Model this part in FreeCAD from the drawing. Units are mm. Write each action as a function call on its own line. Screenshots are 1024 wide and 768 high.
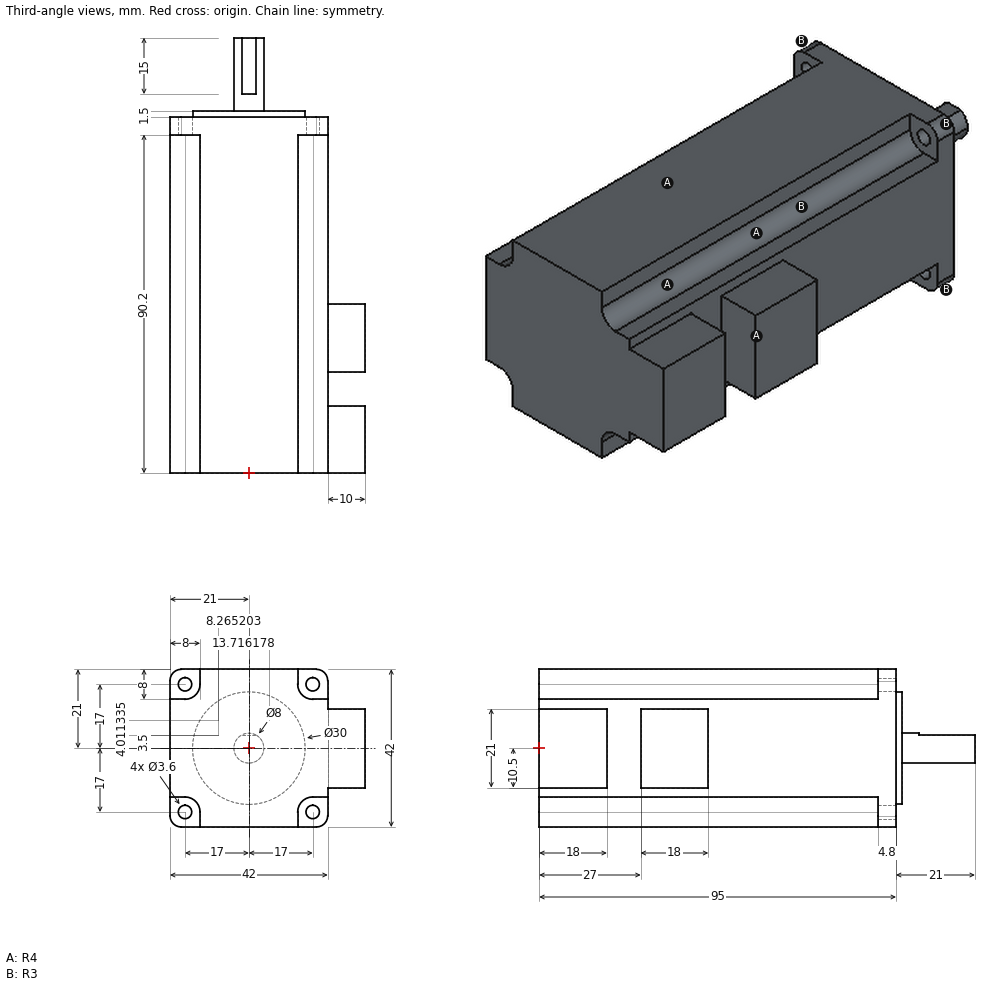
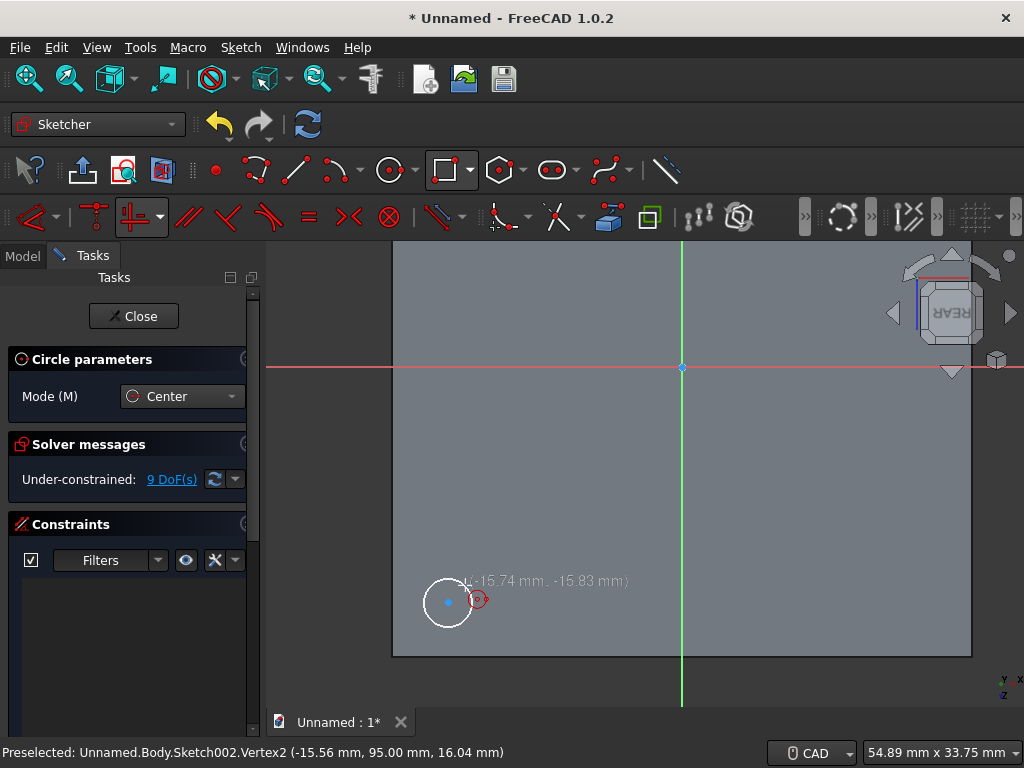
scroll(448, 604, down, 3)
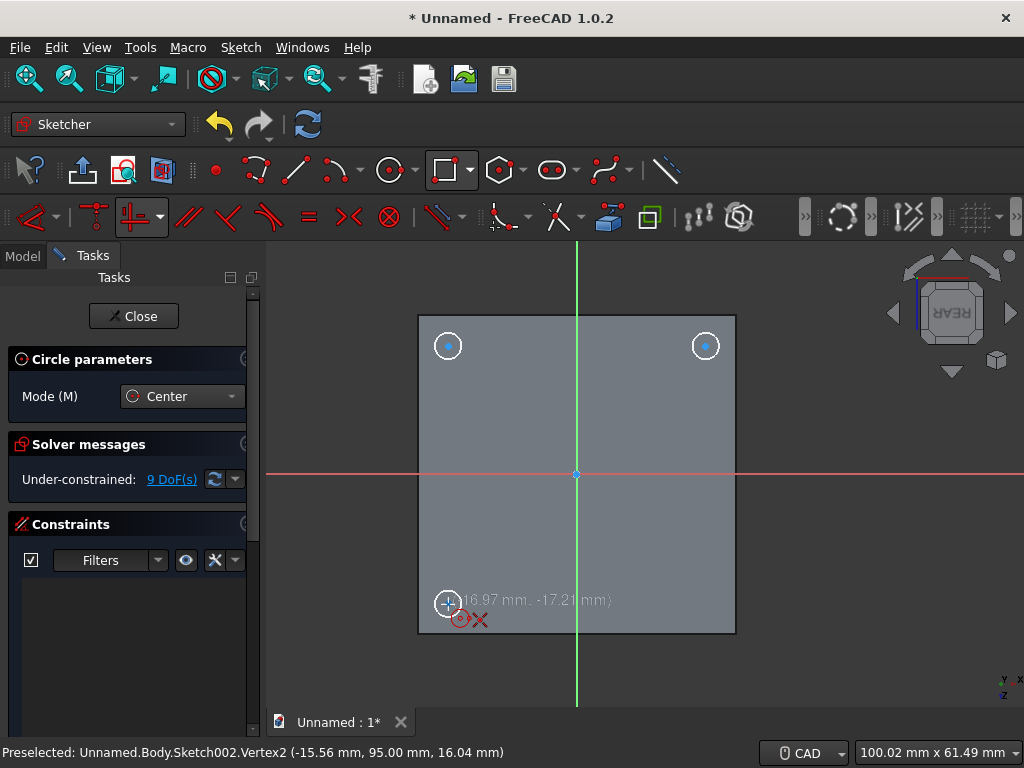
scroll(706, 603, up, 3)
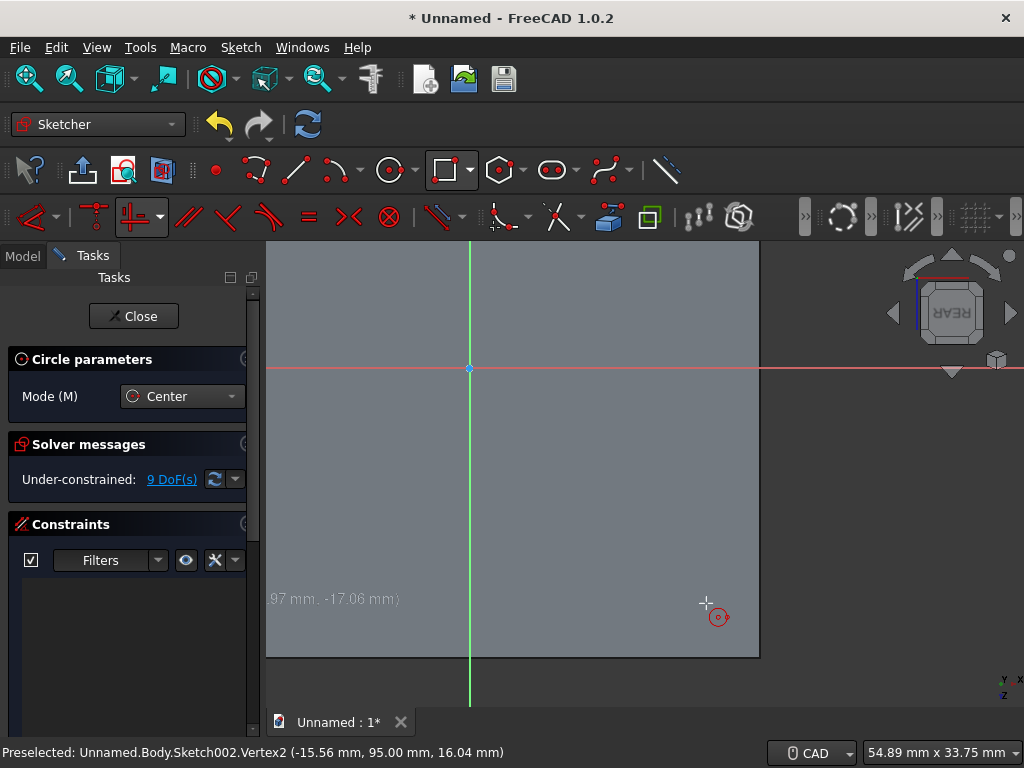
click(705, 603)
click(722, 585)
key(Escape)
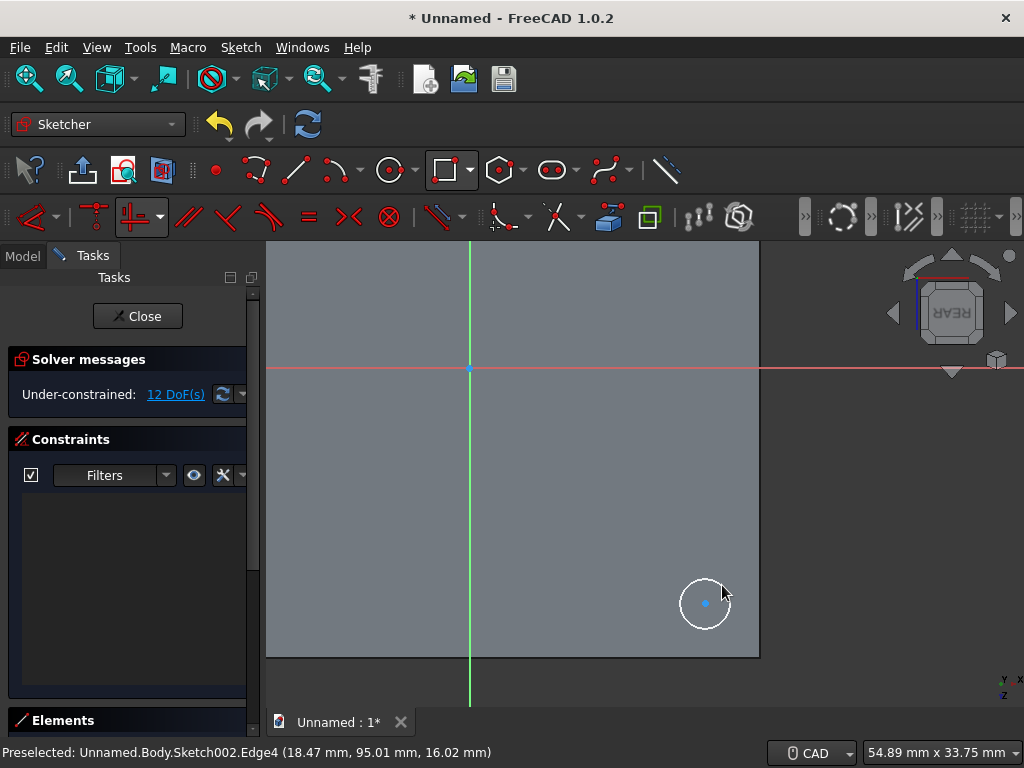
scroll(706, 603, down, 3)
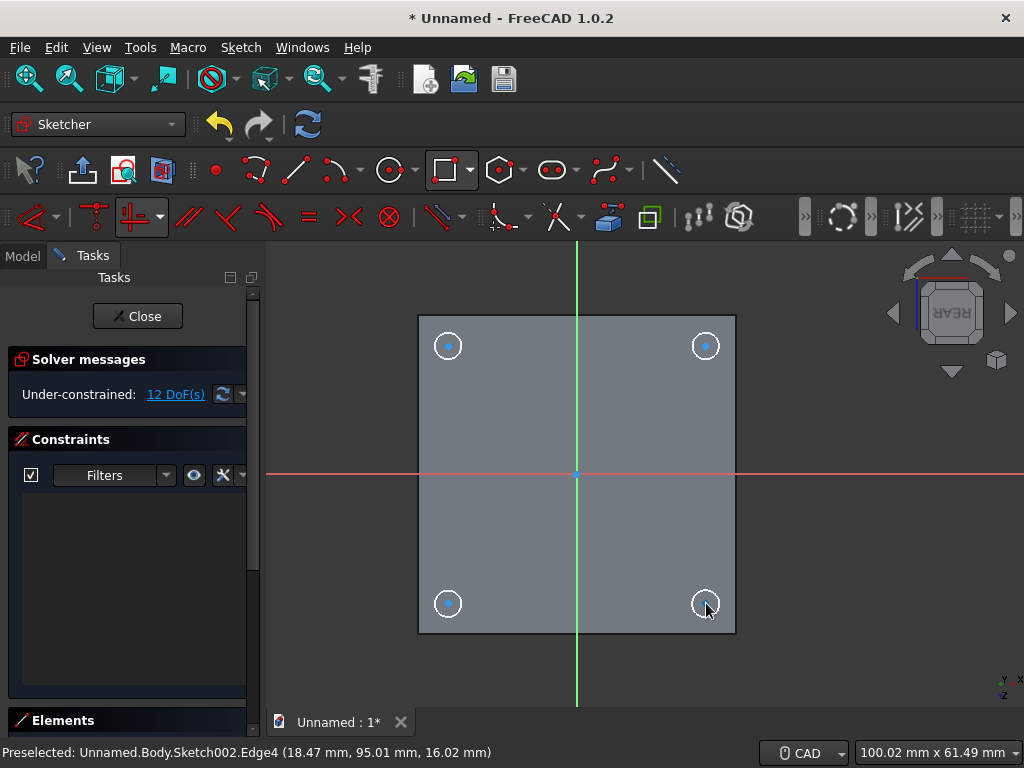
click(457, 337)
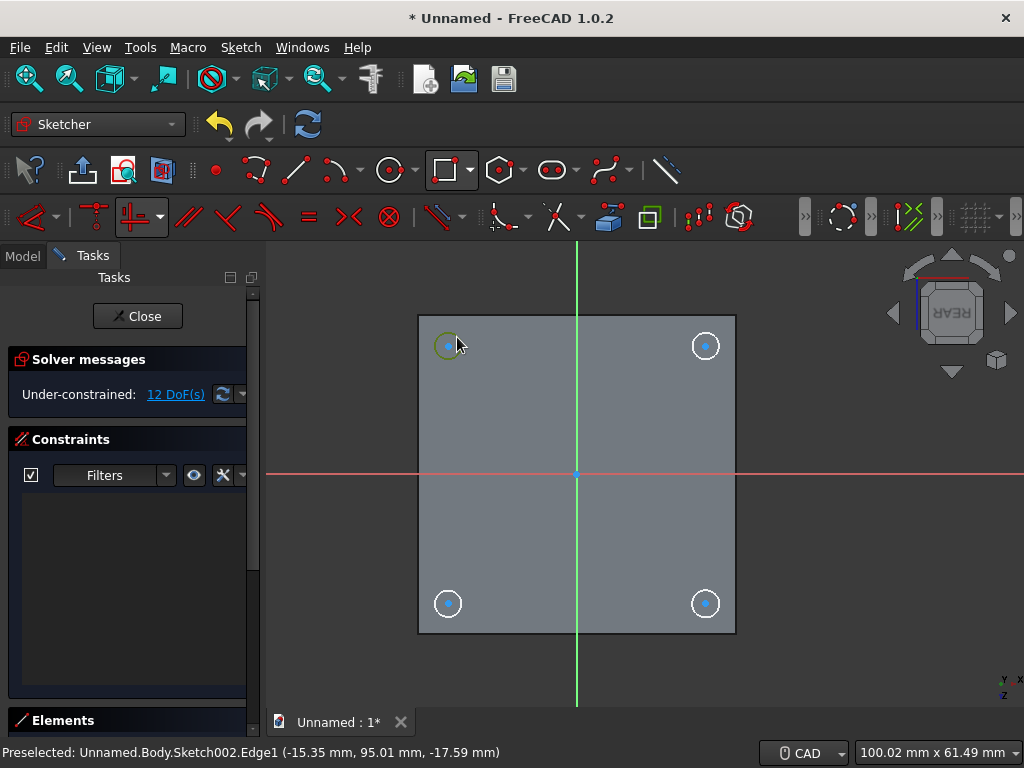
click(715, 337)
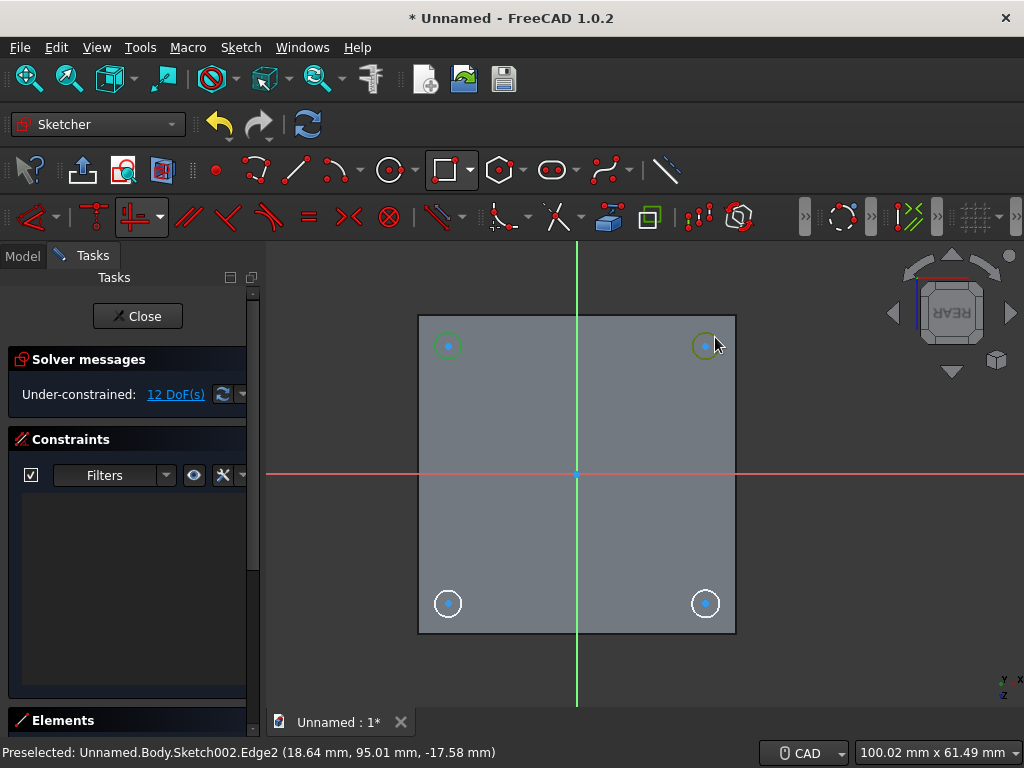
click(457, 594)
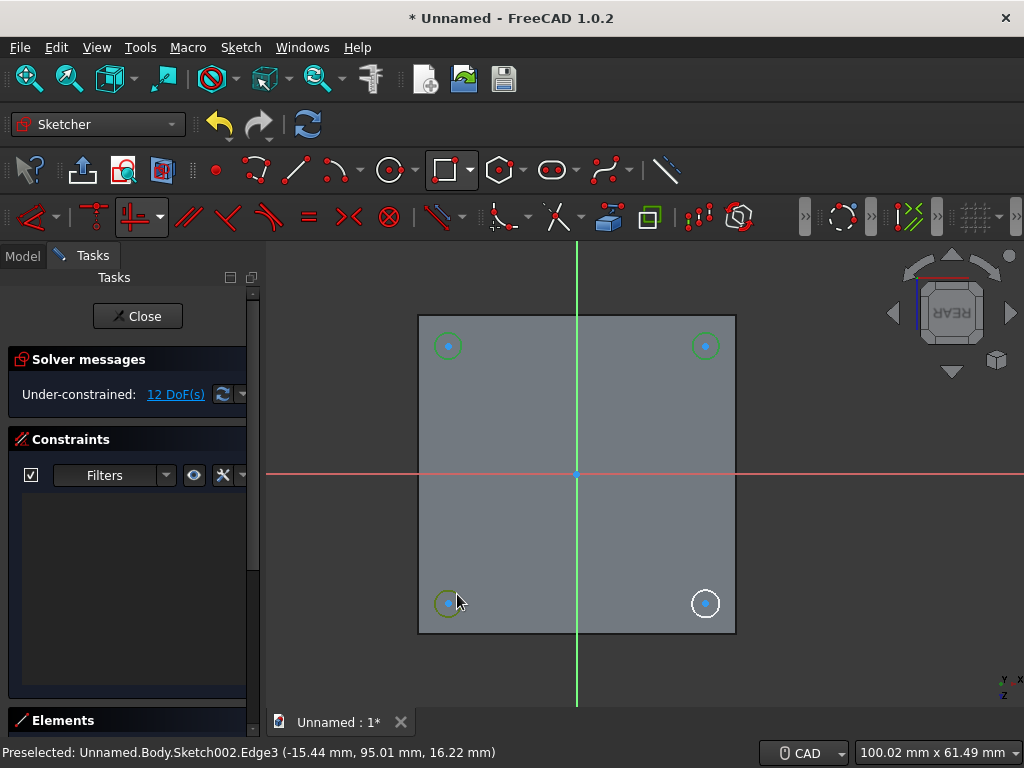
click(715, 594)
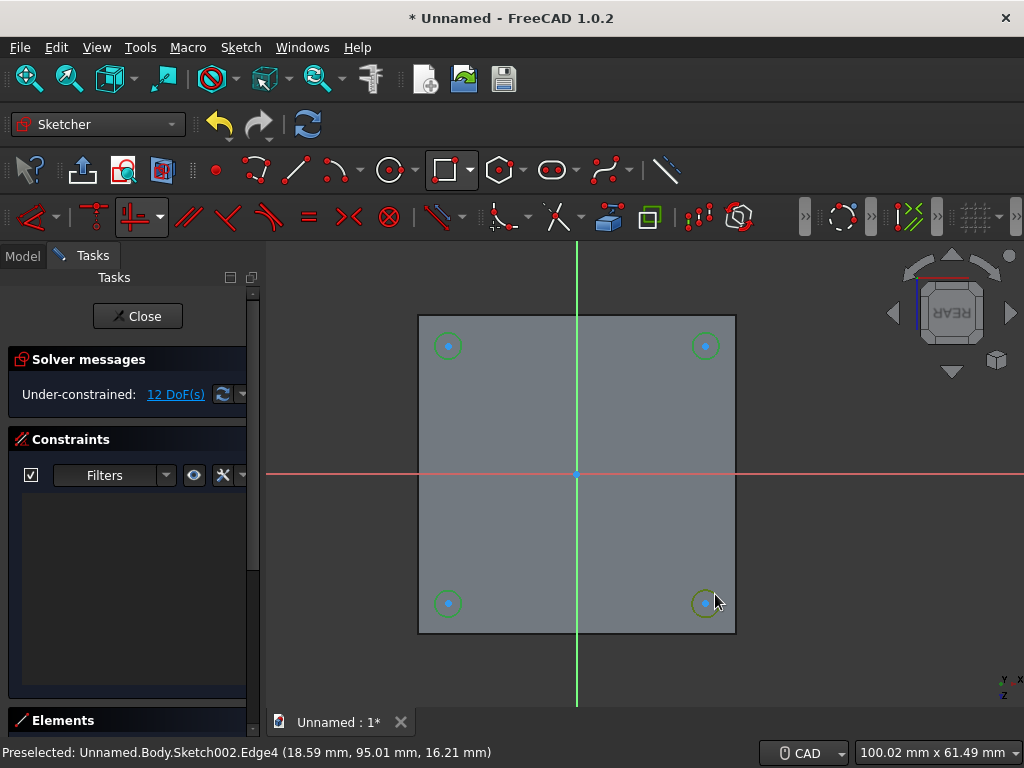
click(310, 218)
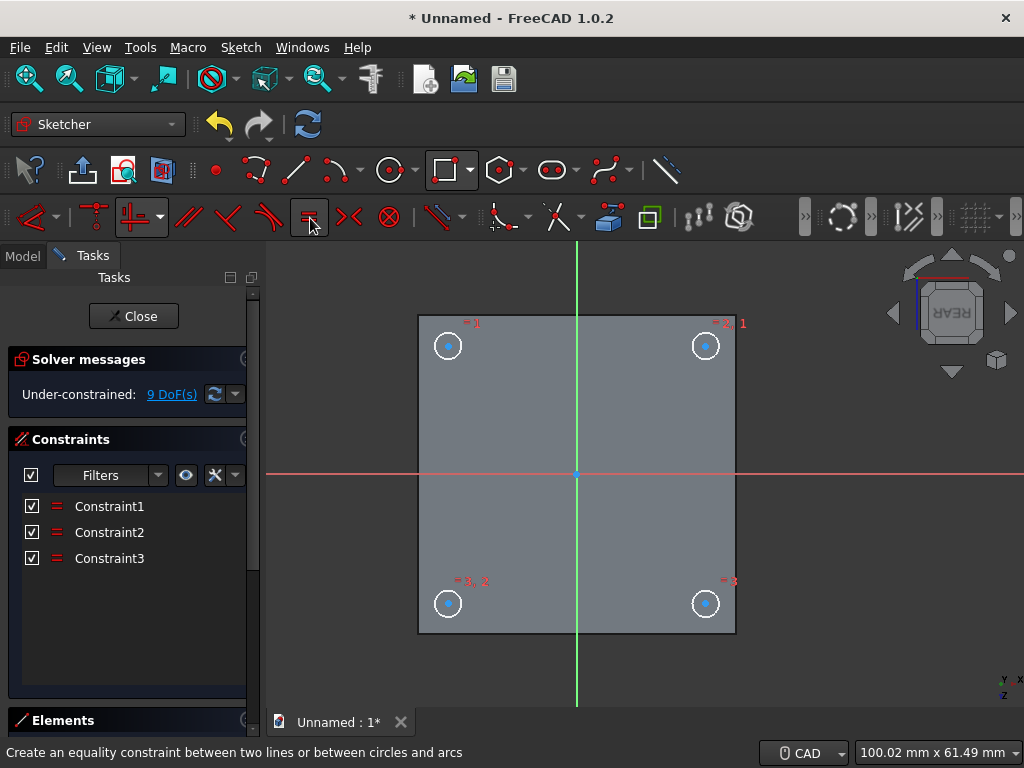
click(448, 346)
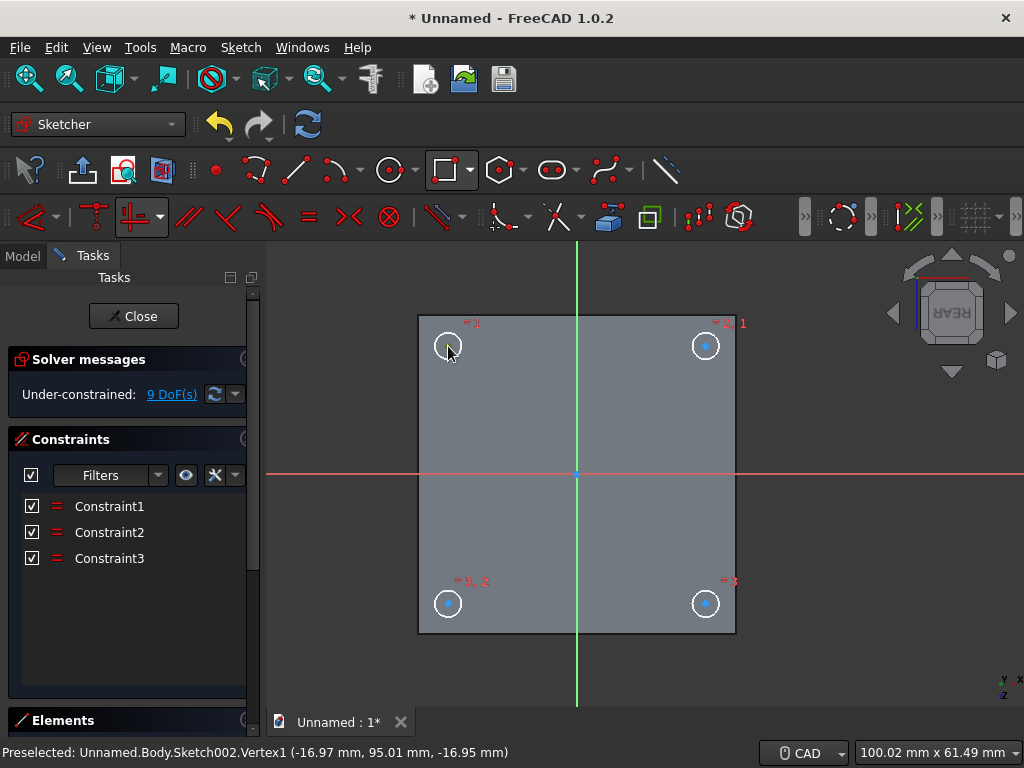
click(706, 346)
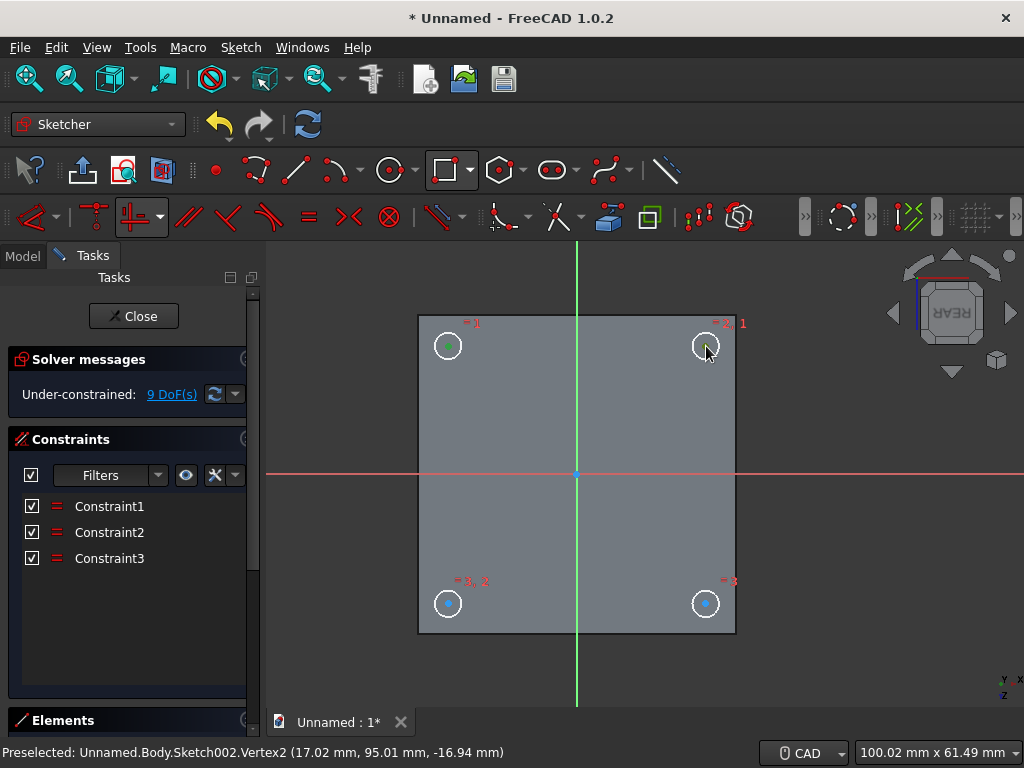
key(h)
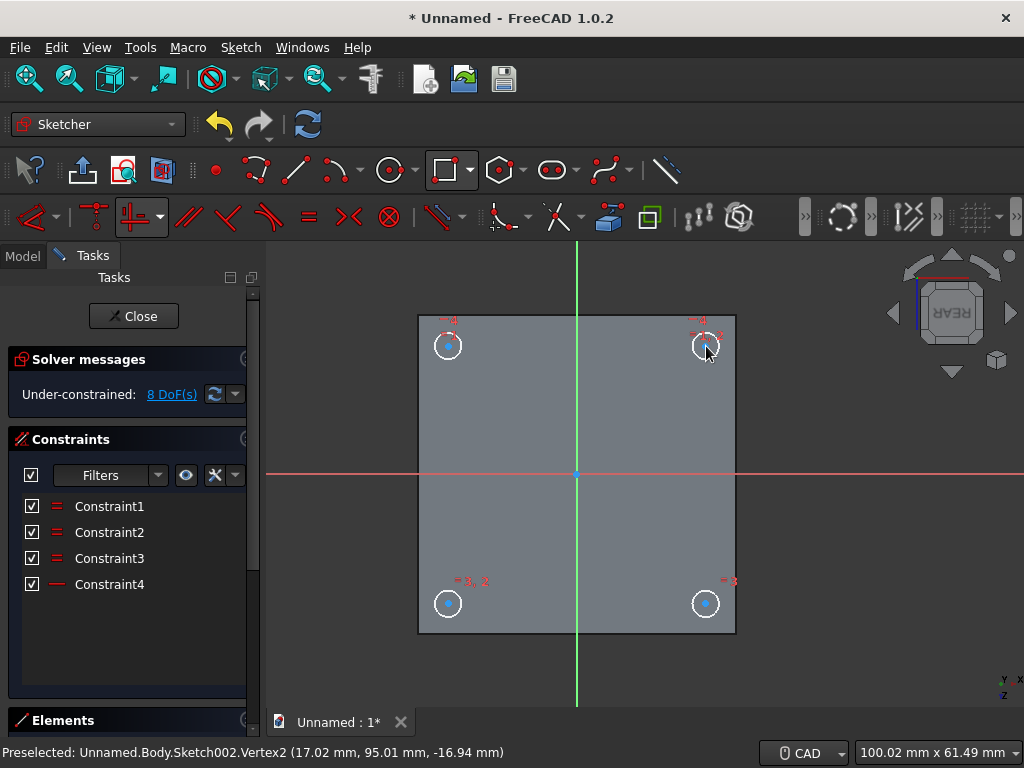
click(448, 346)